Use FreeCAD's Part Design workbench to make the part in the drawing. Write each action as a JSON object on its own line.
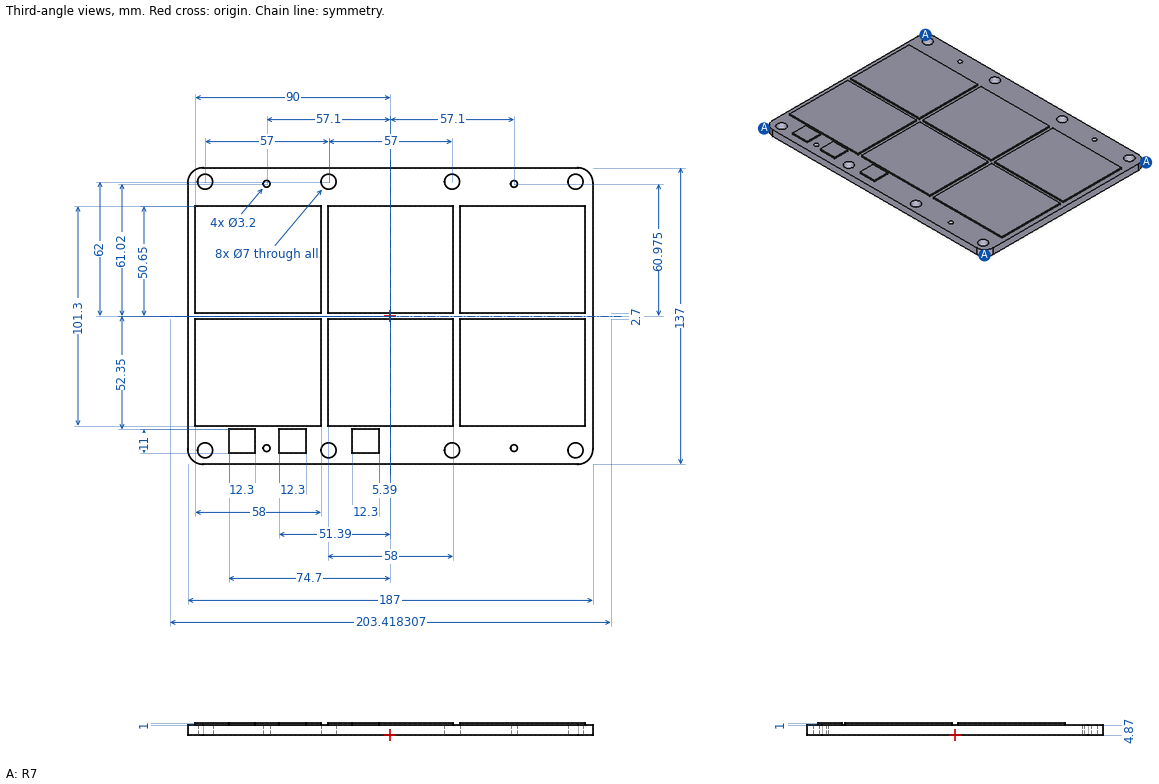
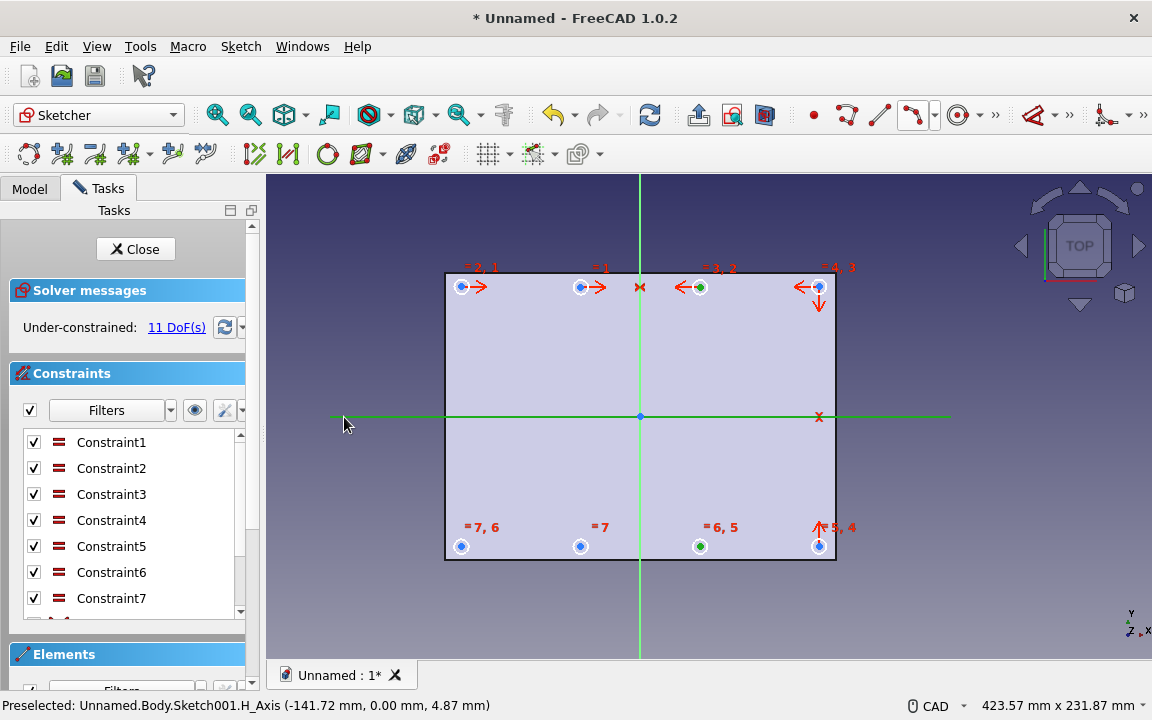
{"action": "key", "text": "s"}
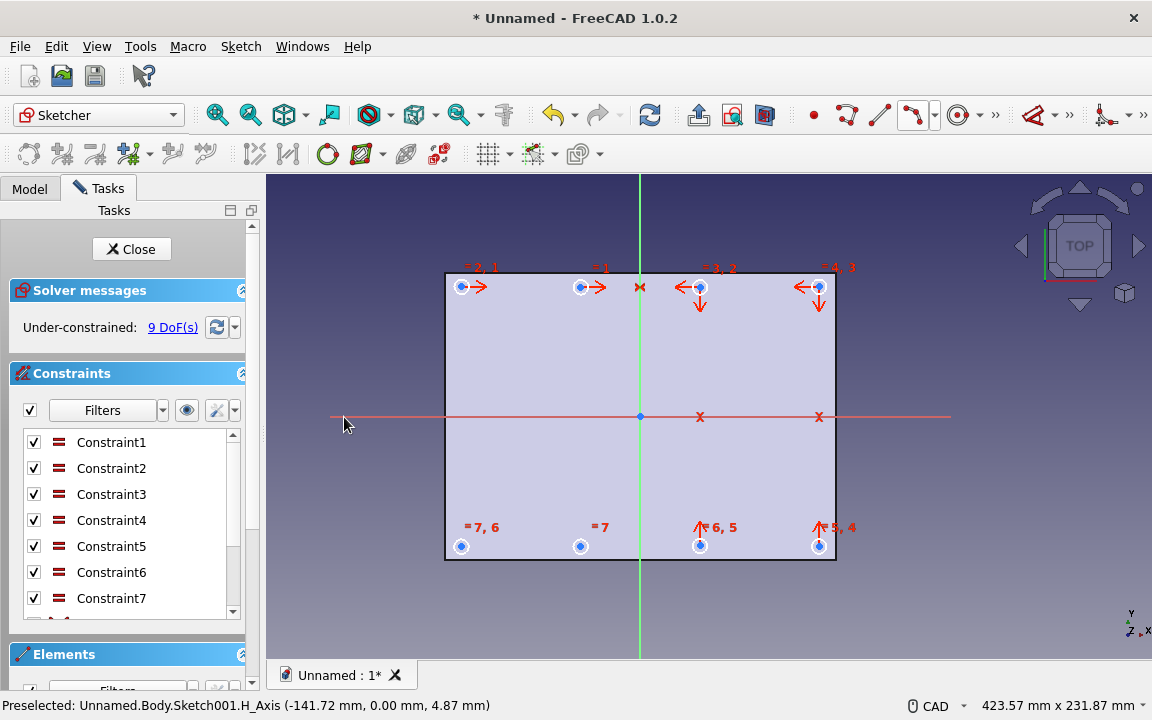
{"action": "left_click", "coordinate": [462, 287]}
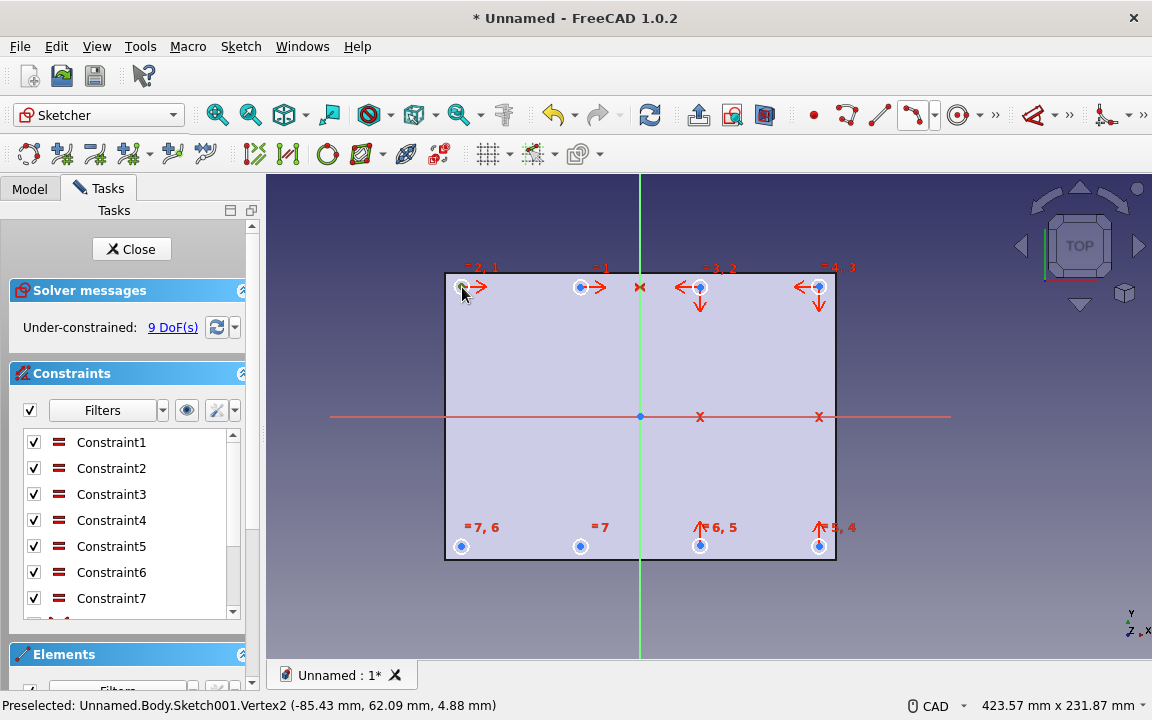
{"action": "left_click", "coordinate": [461, 547]}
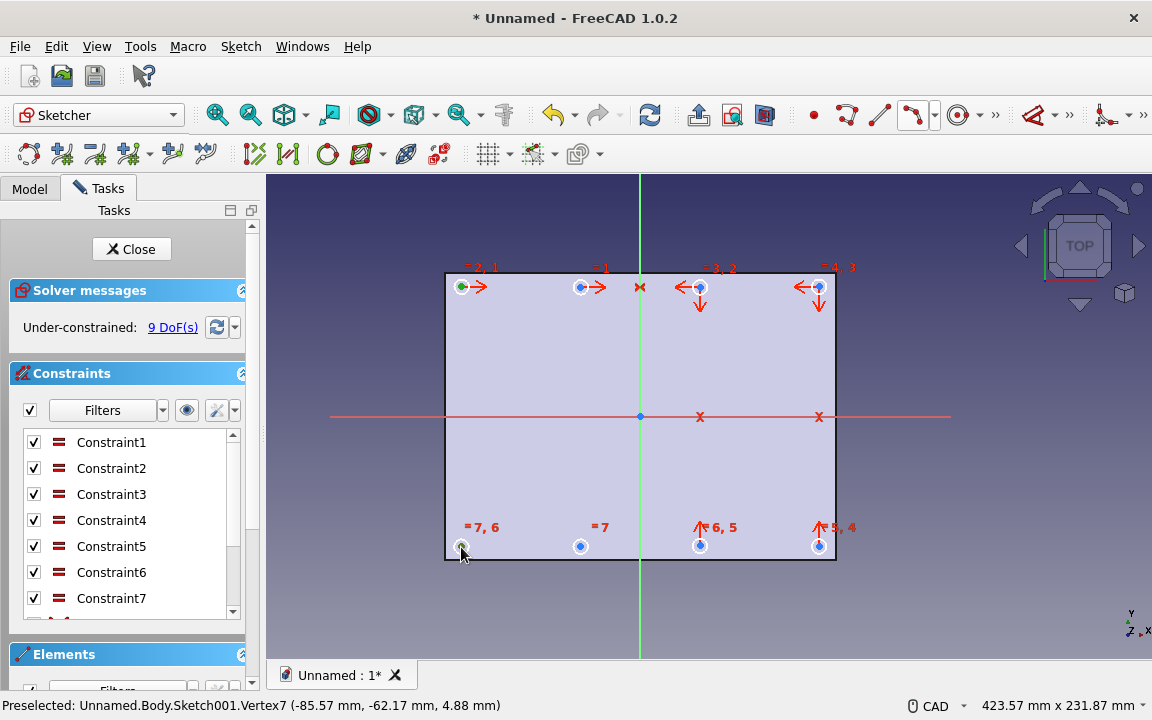
{"action": "left_click", "coordinate": [344, 417]}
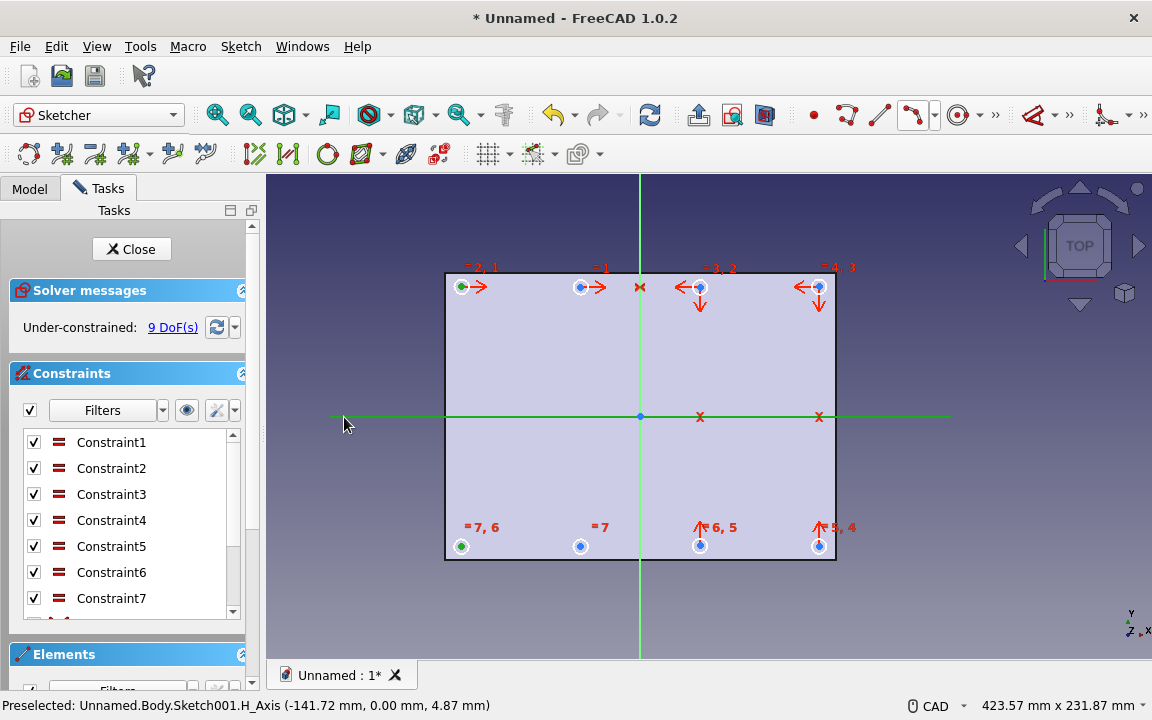
{"action": "key", "text": "s"}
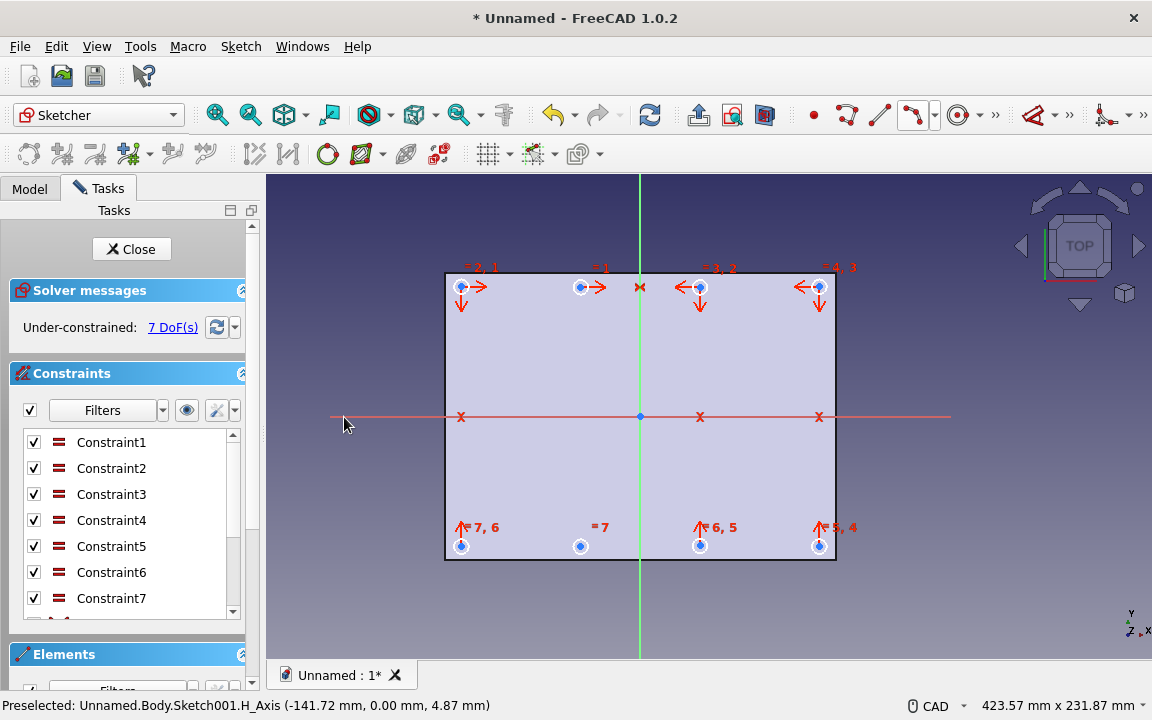
{"action": "left_click", "coordinate": [581, 287]}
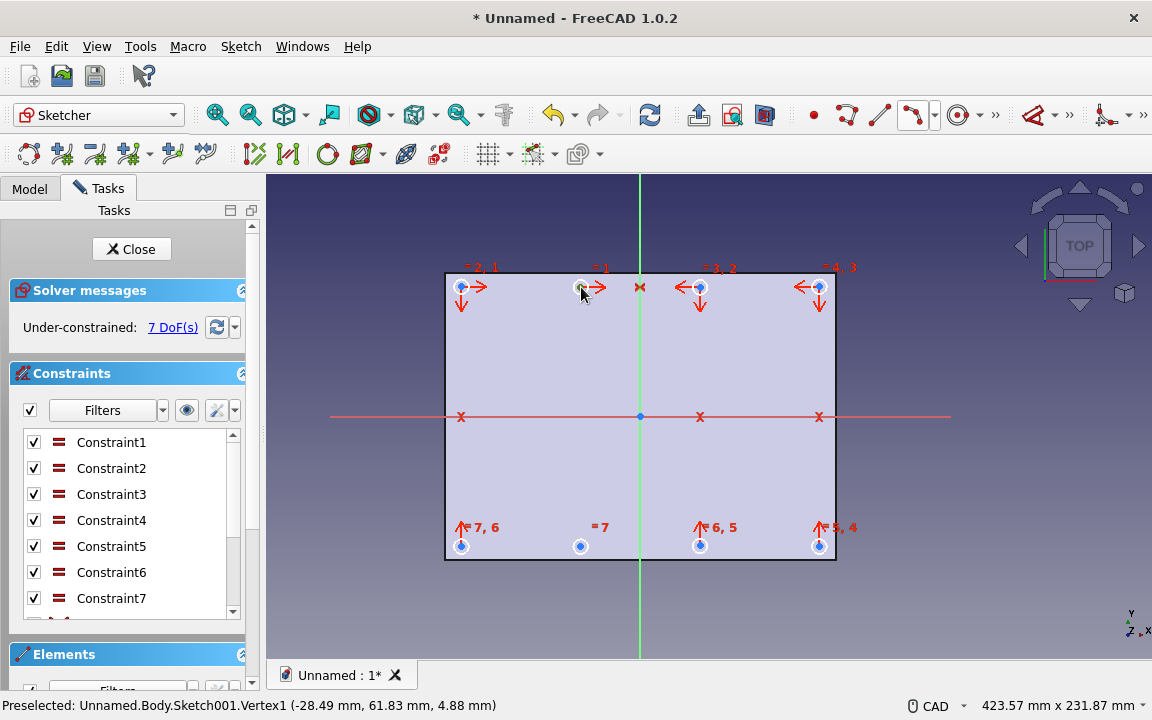
{"action": "left_click", "coordinate": [581, 547]}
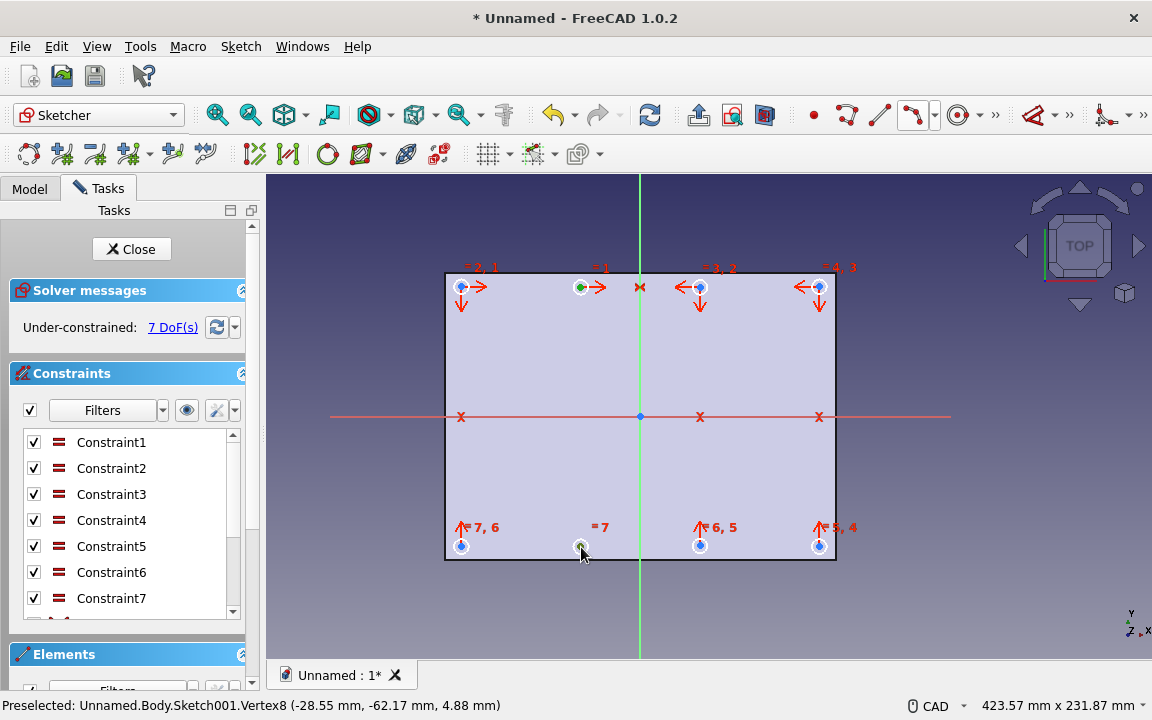
{"action": "left_click", "coordinate": [344, 417]}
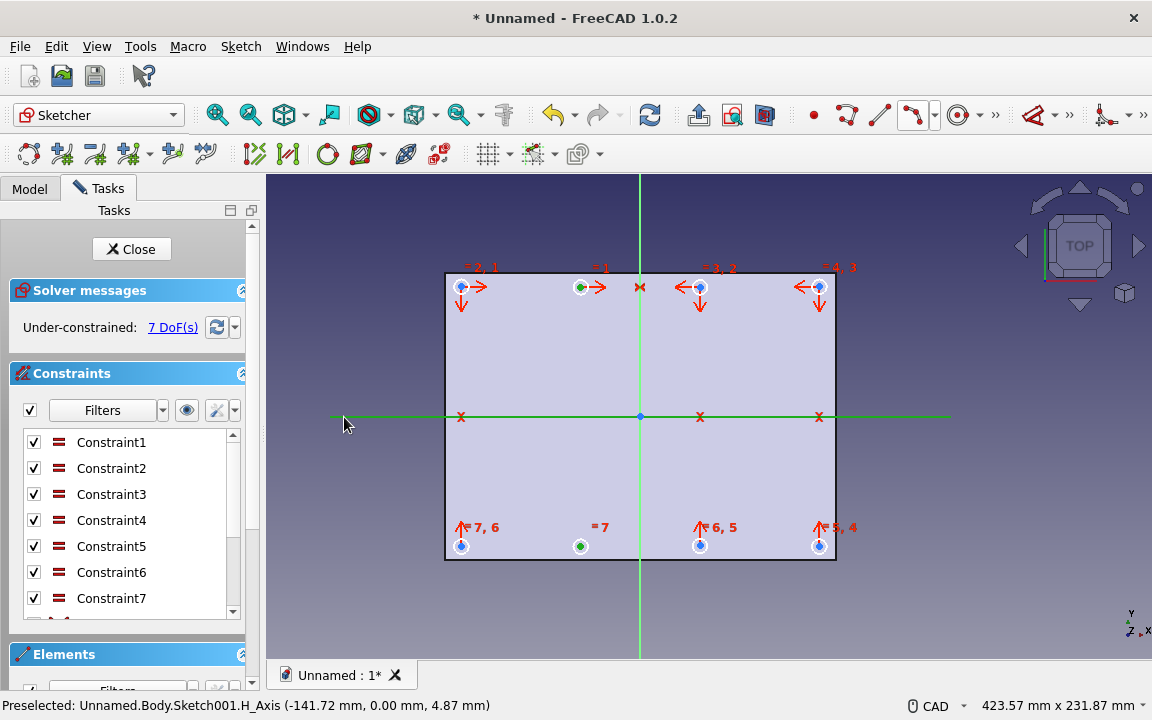
{"action": "key", "text": "s"}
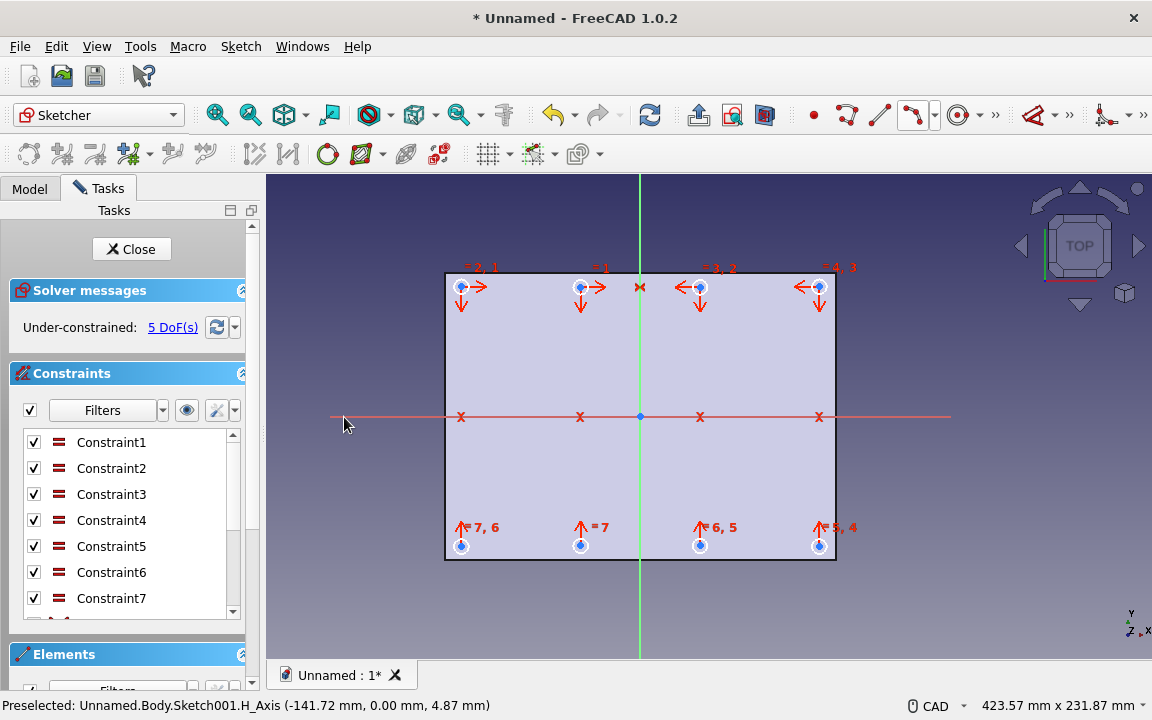
{"action": "key", "text": "d"}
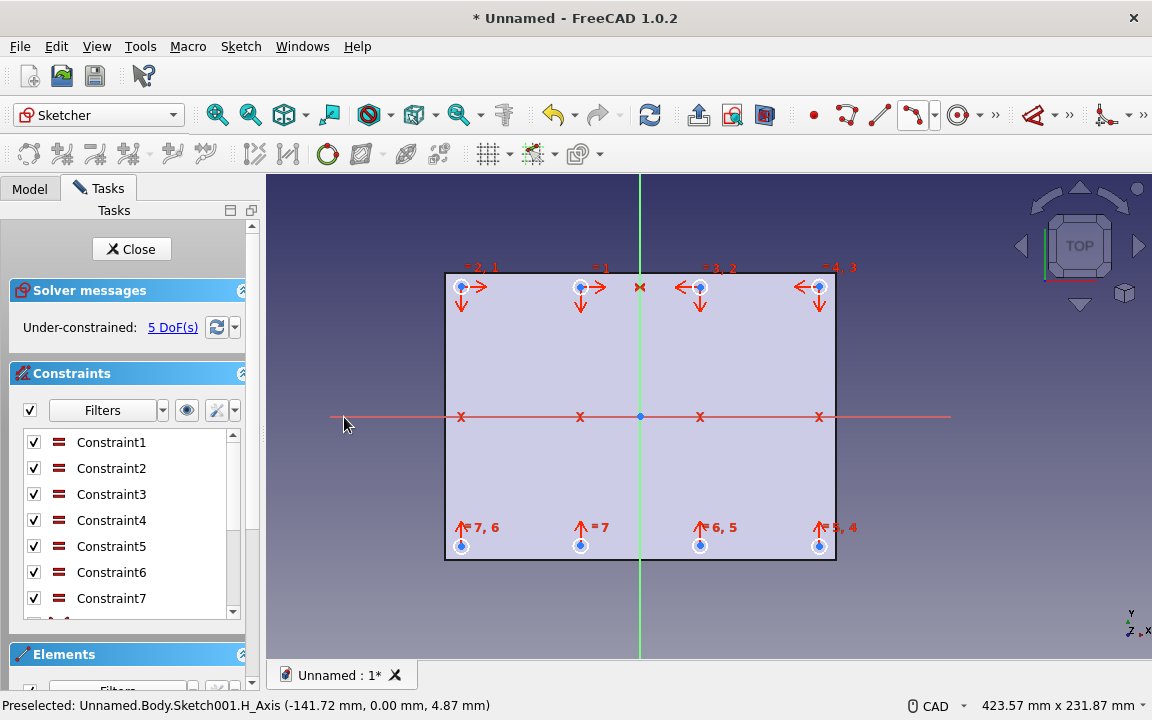
{"action": "scroll", "coordinate": [586, 292], "scroll_direction": "up", "scroll_amount": 5}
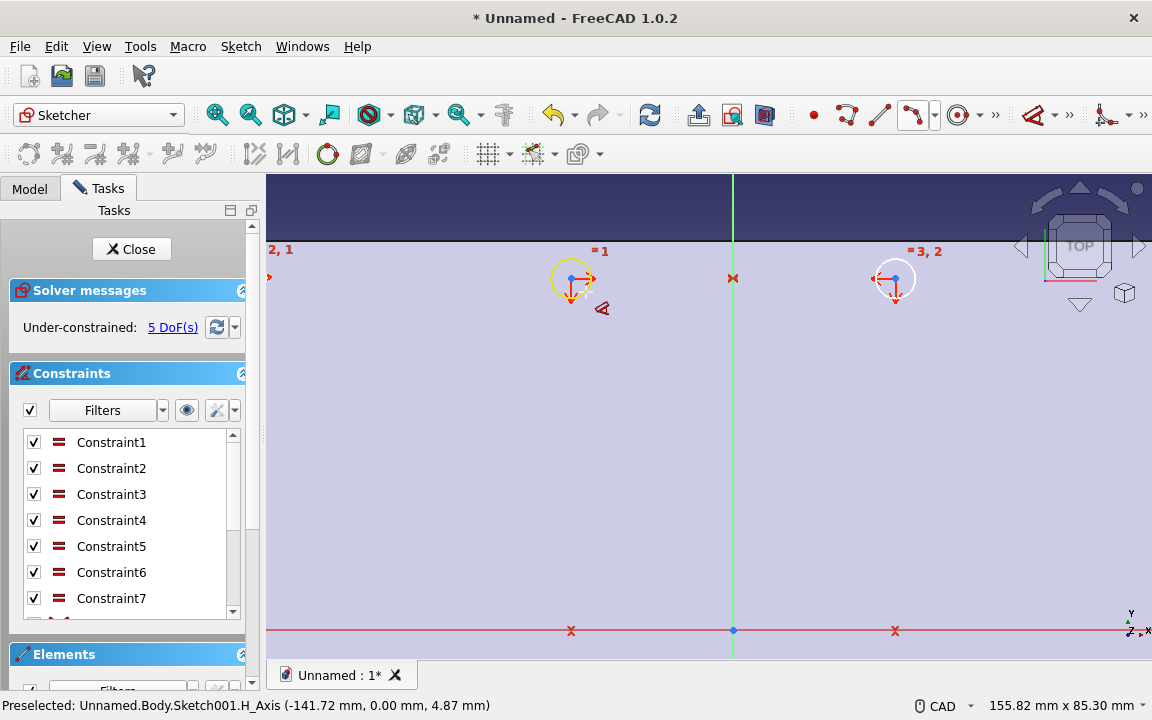
{"action": "left_click", "coordinate": [585, 293]}
{"action": "left_click", "coordinate": [607, 316]}